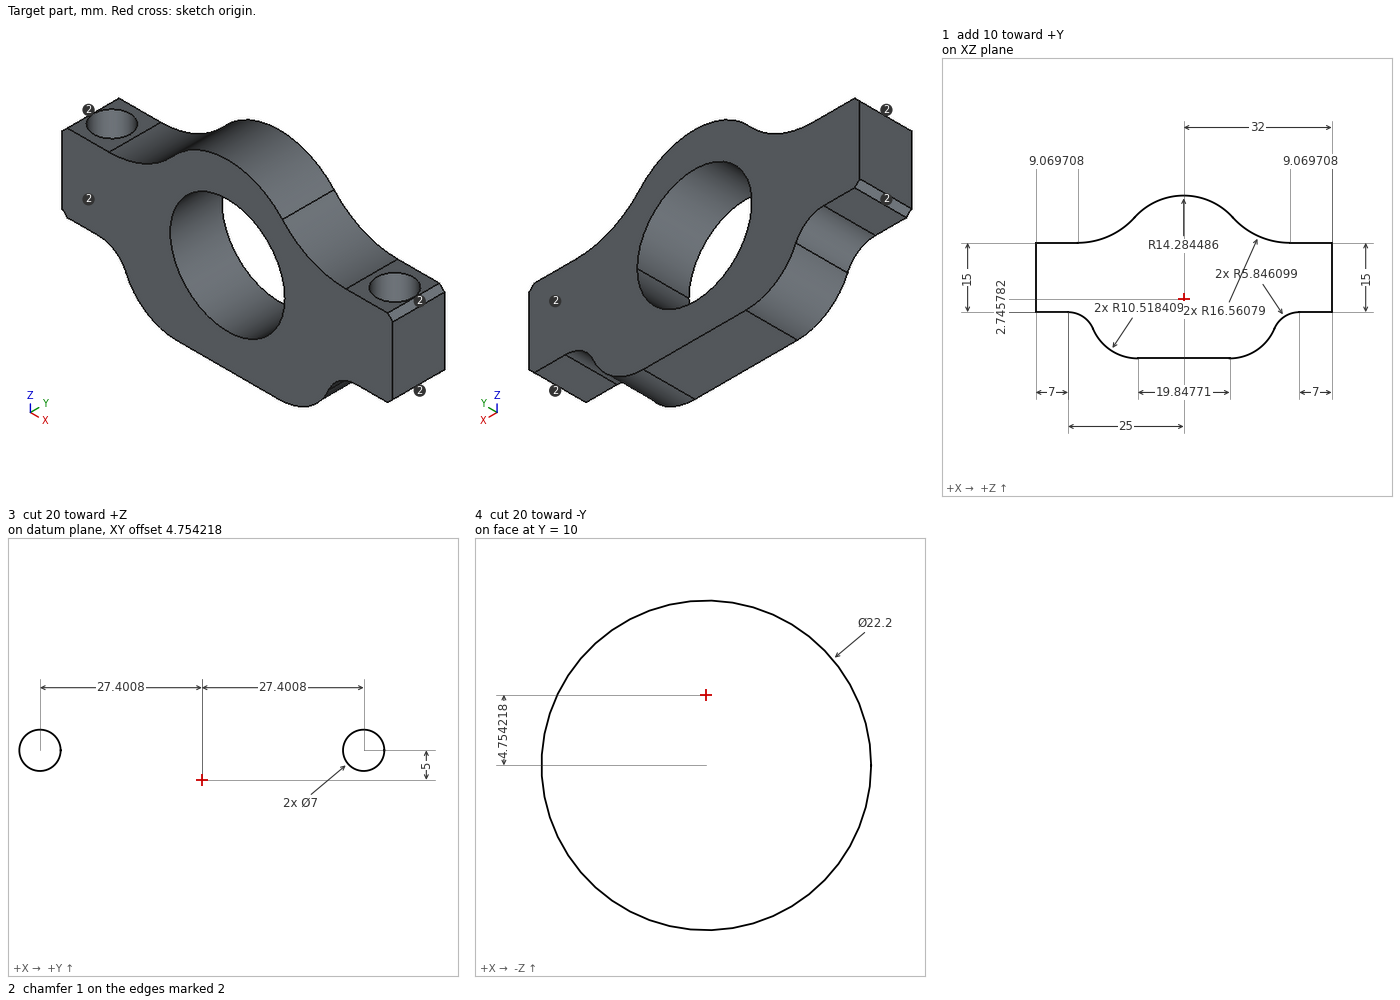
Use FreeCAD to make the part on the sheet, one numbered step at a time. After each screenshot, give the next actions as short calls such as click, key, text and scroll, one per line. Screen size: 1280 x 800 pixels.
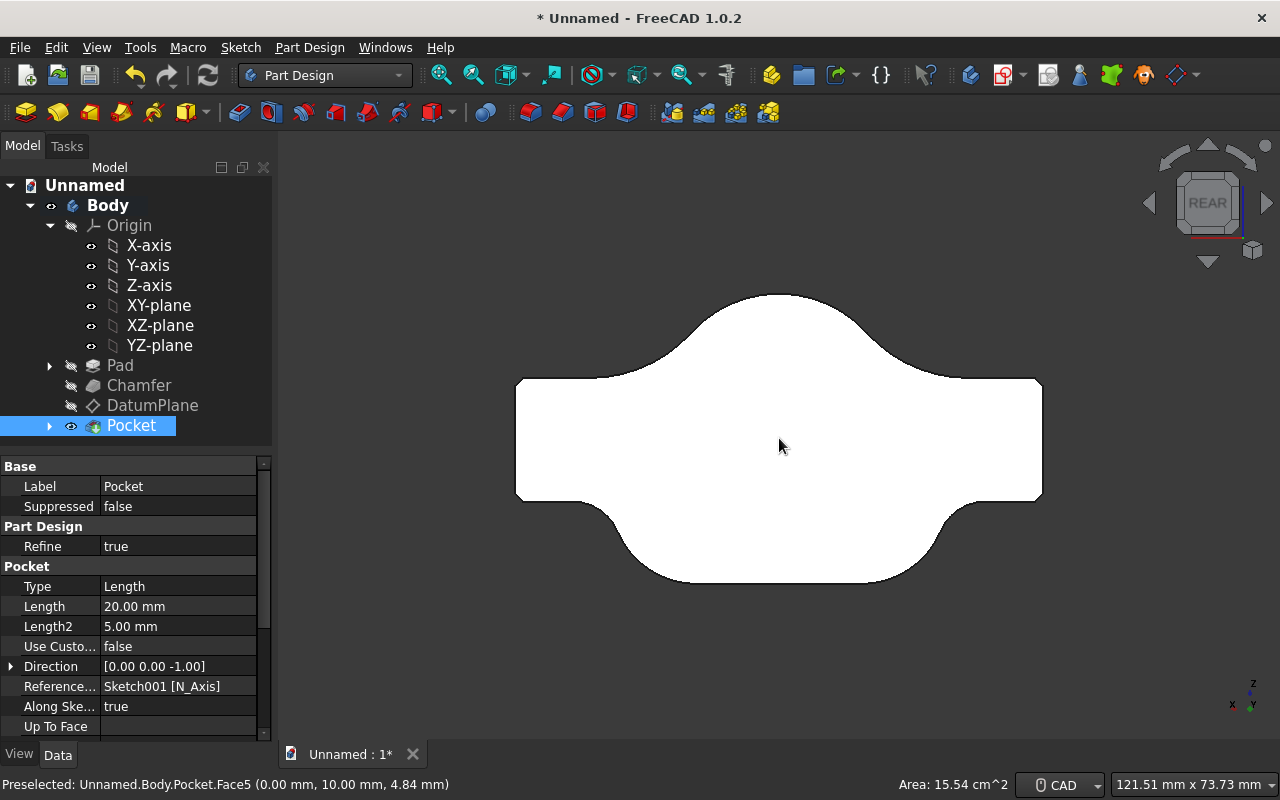
click(1004, 76)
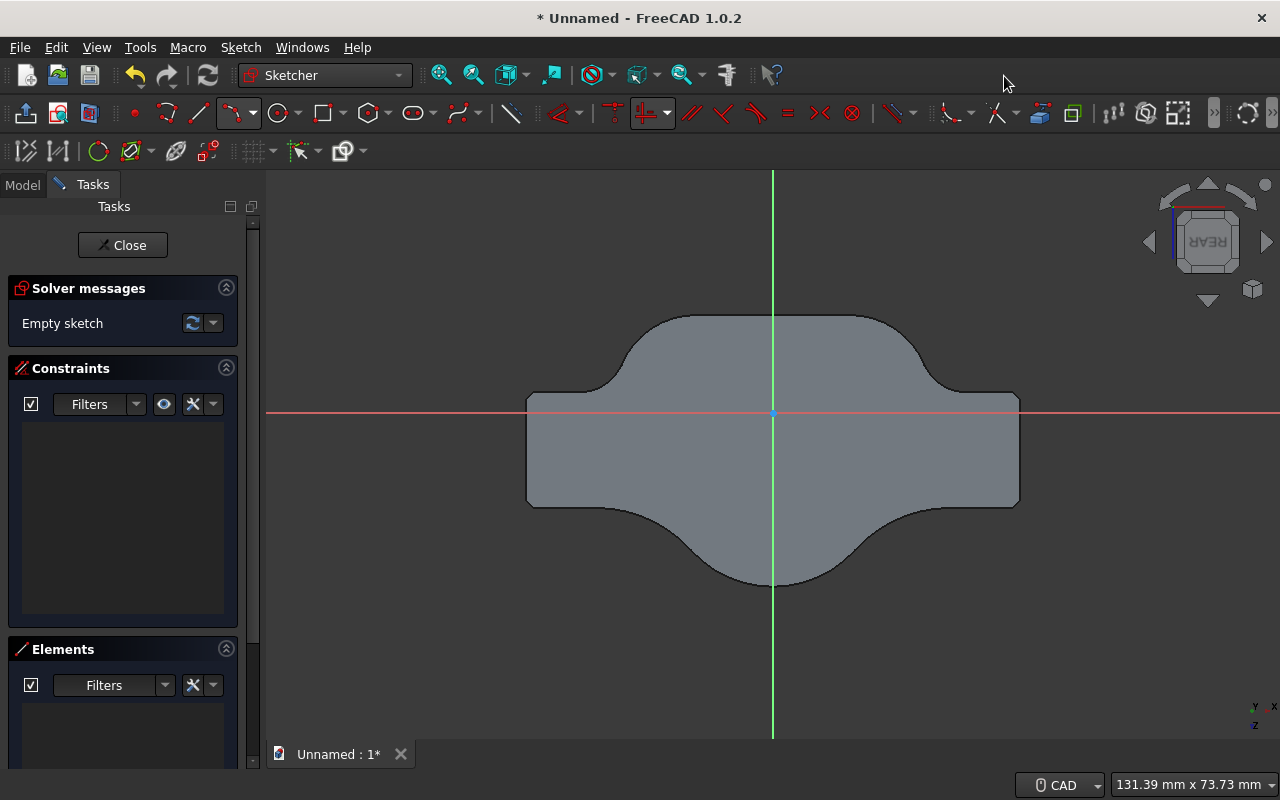
scroll(829, 446, up, 4)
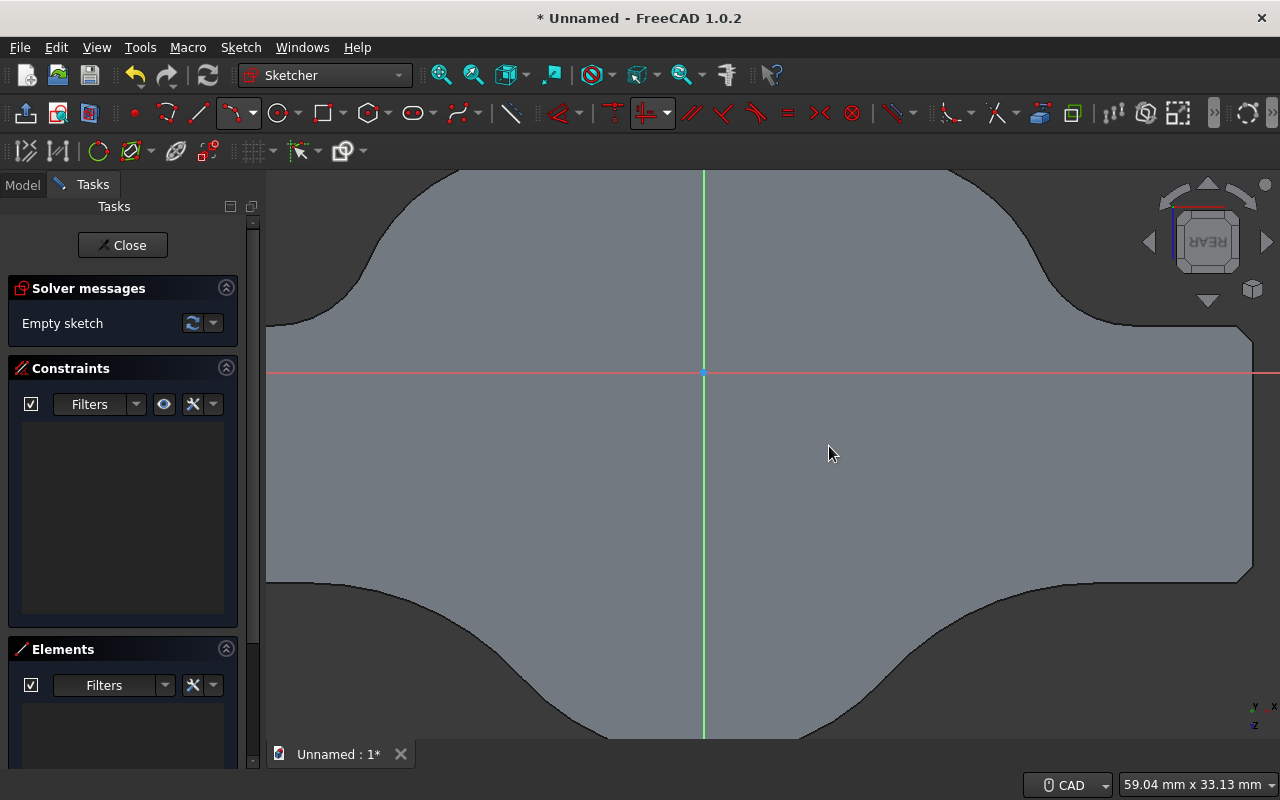
click(278, 114)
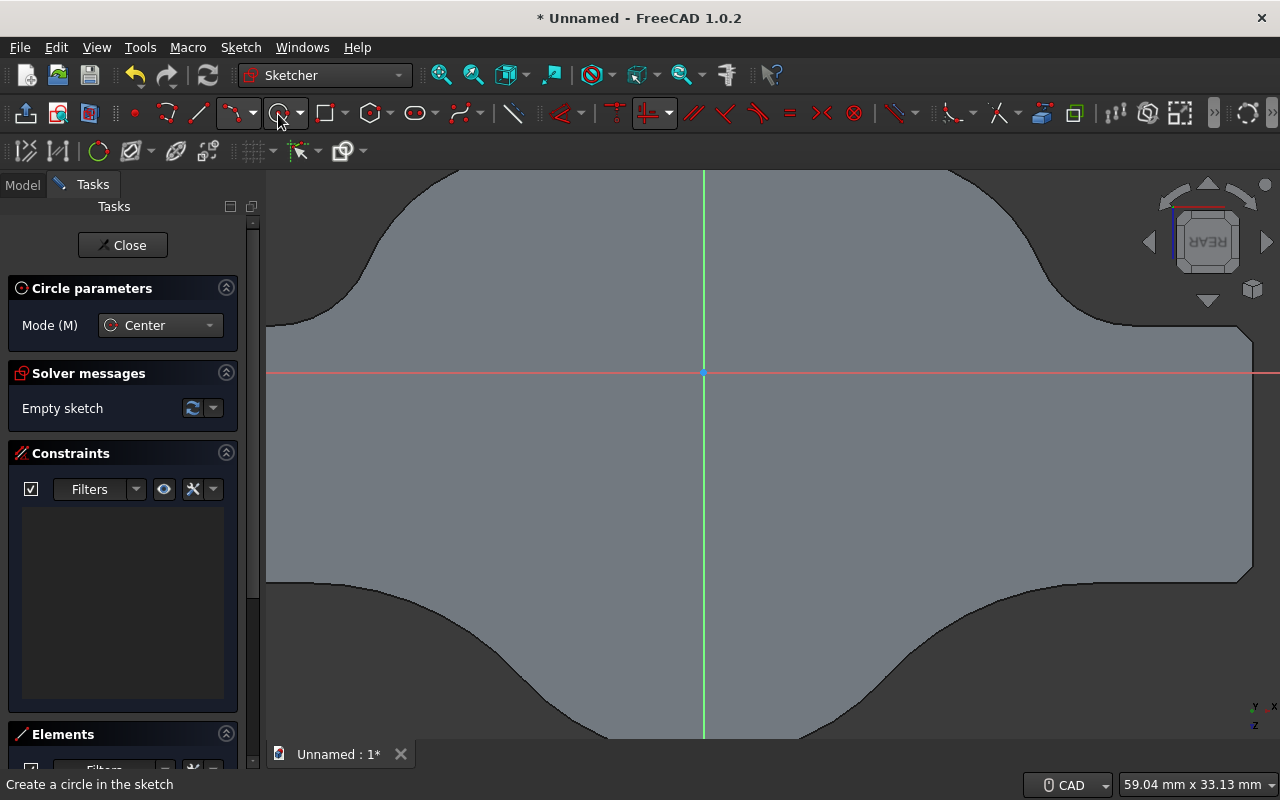
click(704, 454)
move(838, 320)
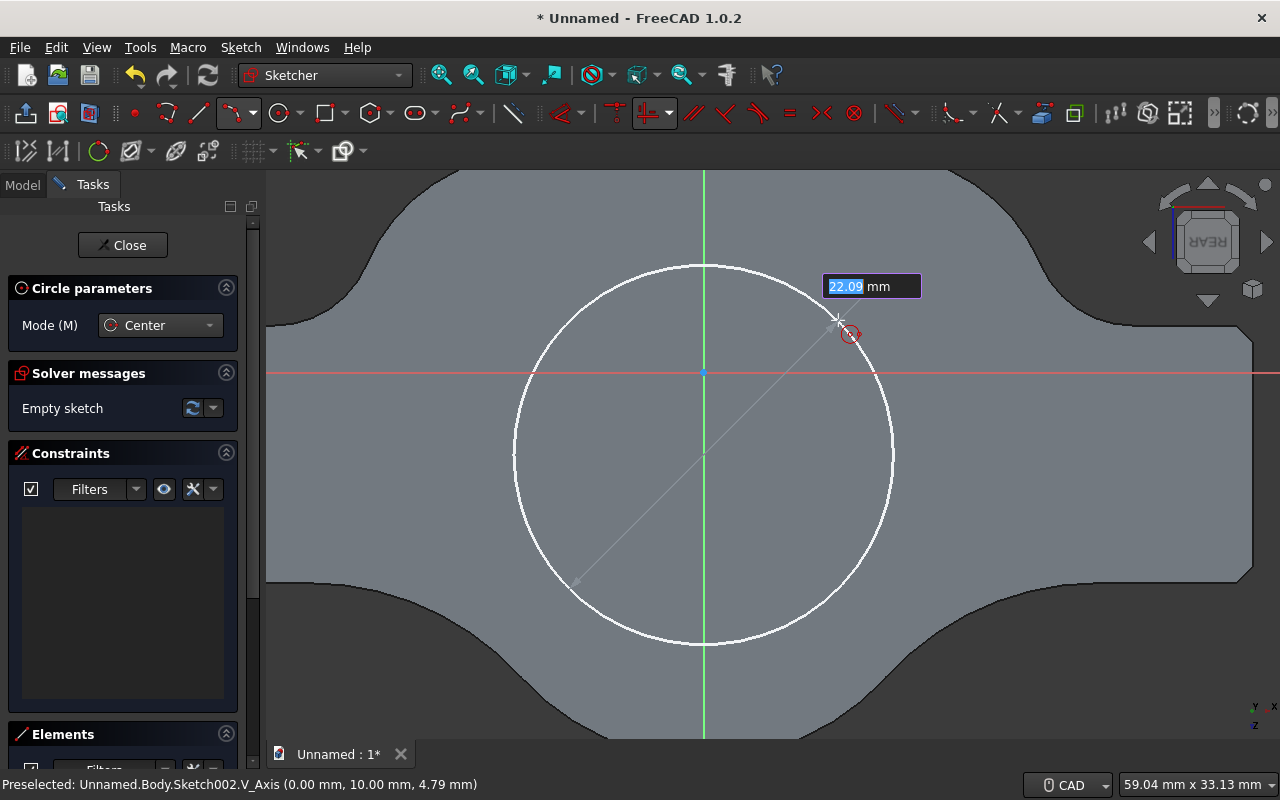
text(22.2)
key(Return)
key(Escape)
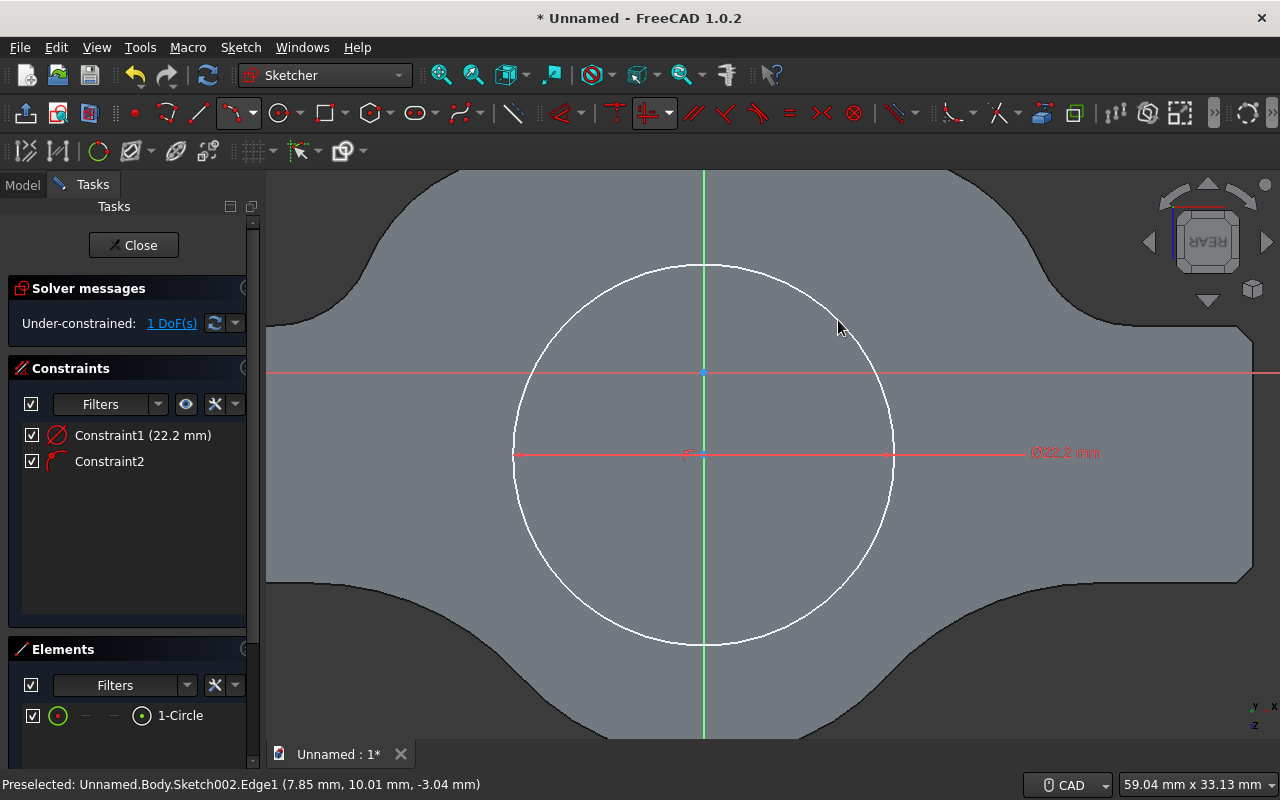
click(560, 114)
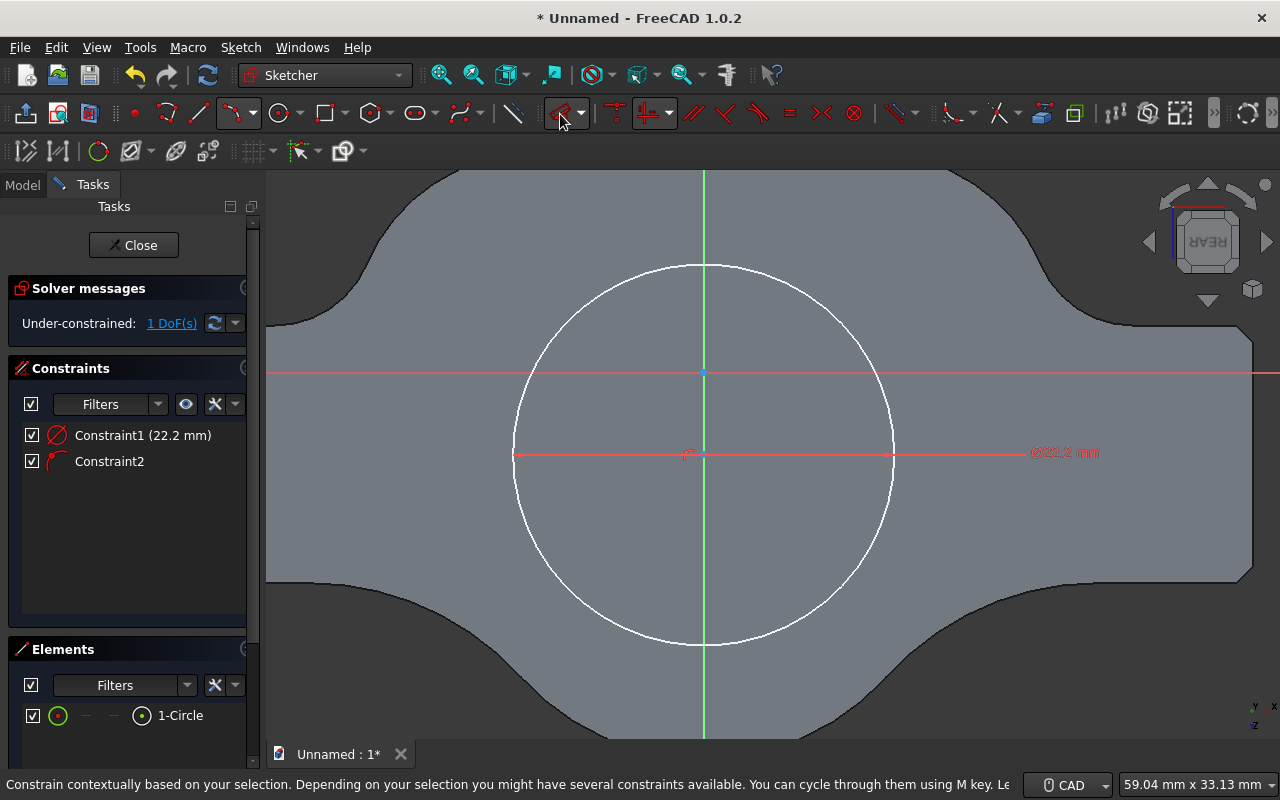
click(704, 455)
click(738, 414)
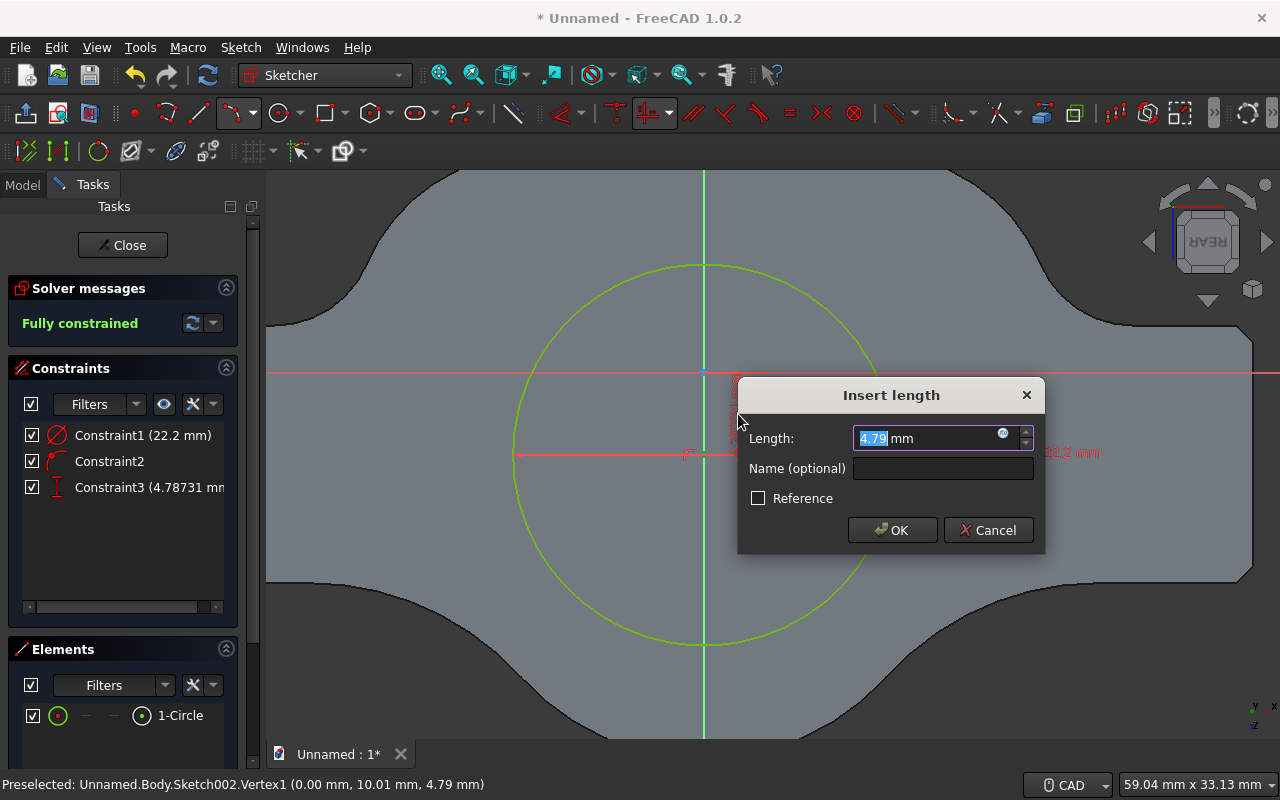
text(4.754218)
key(Return)
key(Escape)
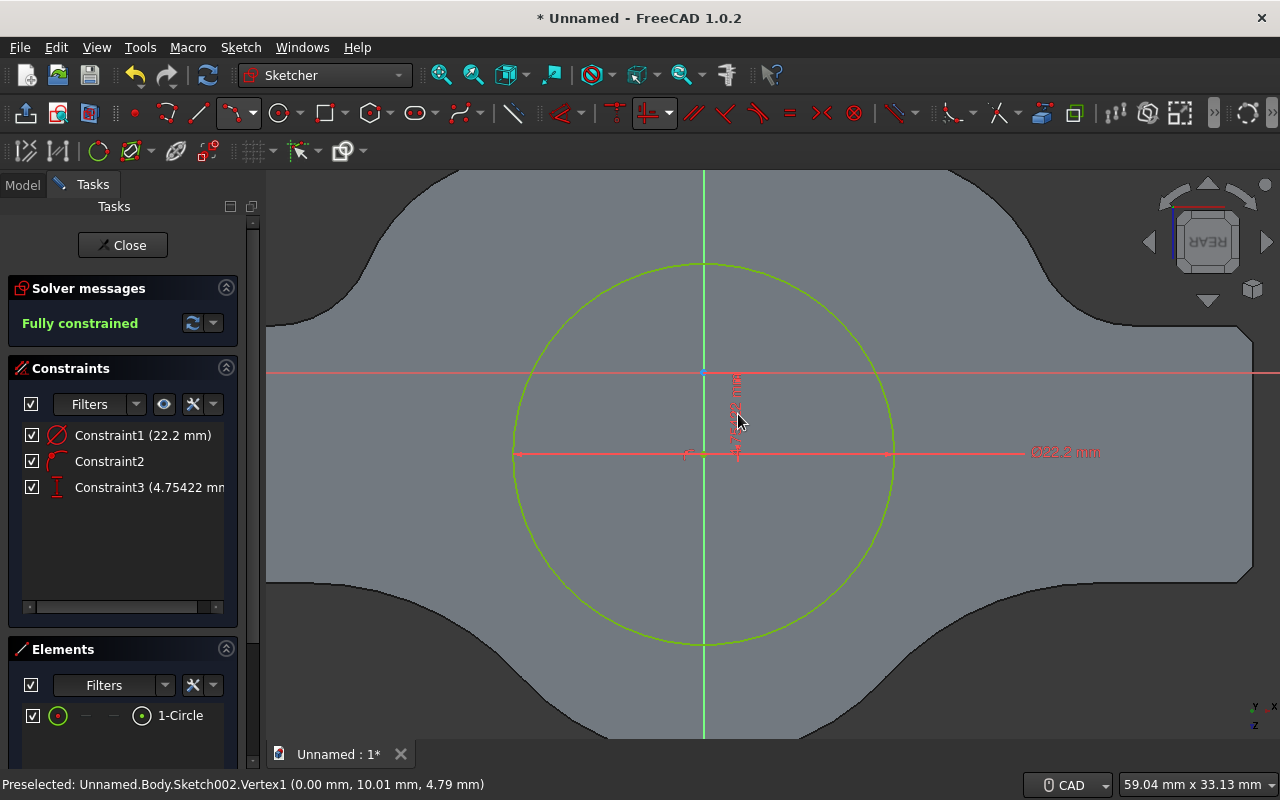
click(123, 245)